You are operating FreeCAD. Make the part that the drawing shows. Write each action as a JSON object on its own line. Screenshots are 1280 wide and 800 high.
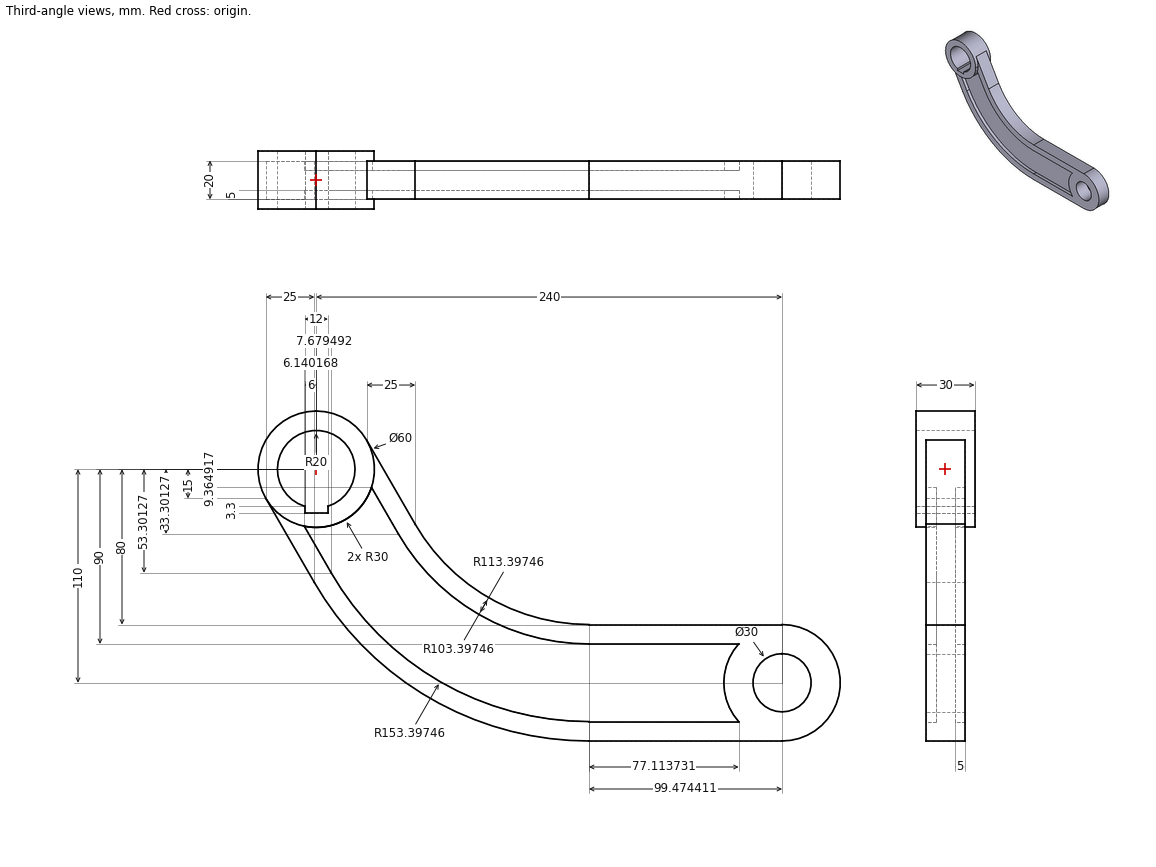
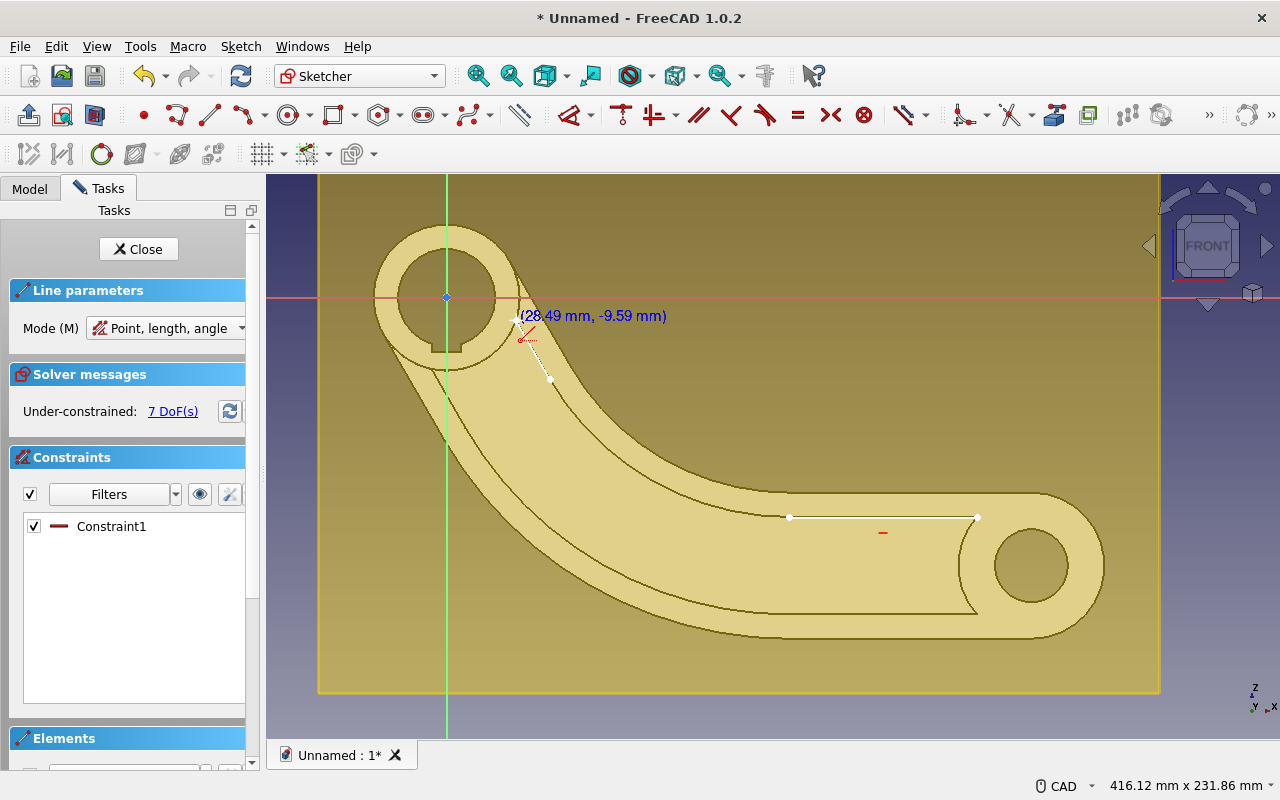
{"action": "left_click", "coordinate": [432, 369]}
{"action": "left_click", "coordinate": [465, 428]}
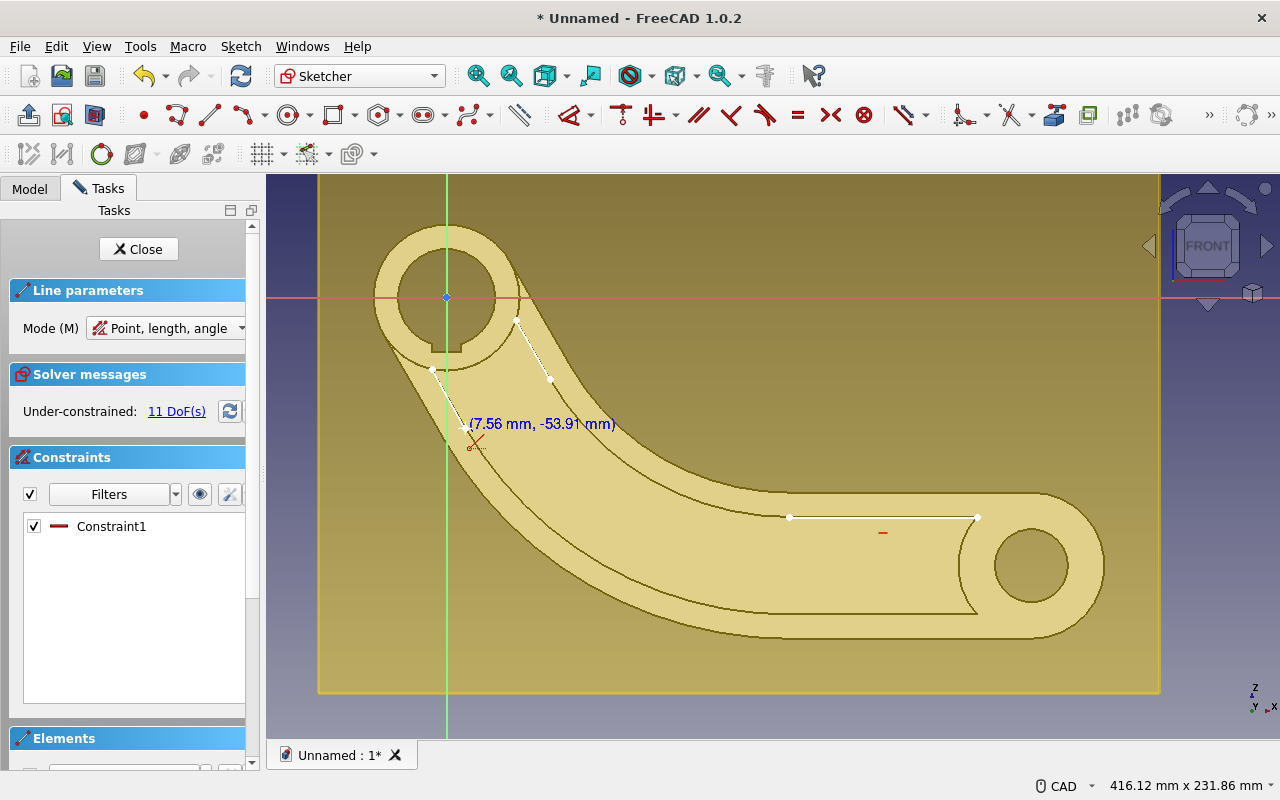
{"action": "left_click", "coordinate": [789, 614]}
{"action": "left_click", "coordinate": [977, 614]}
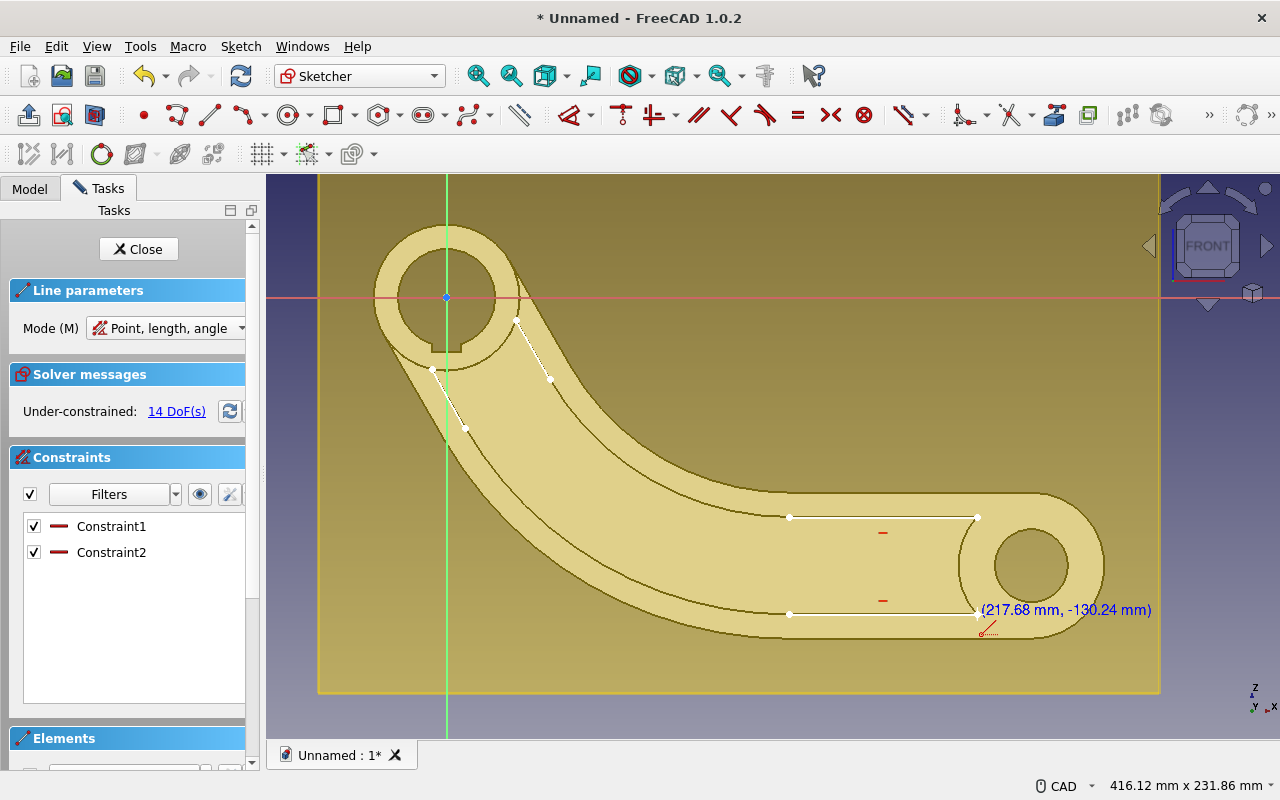
{"action": "left_click", "coordinate": [242, 116]}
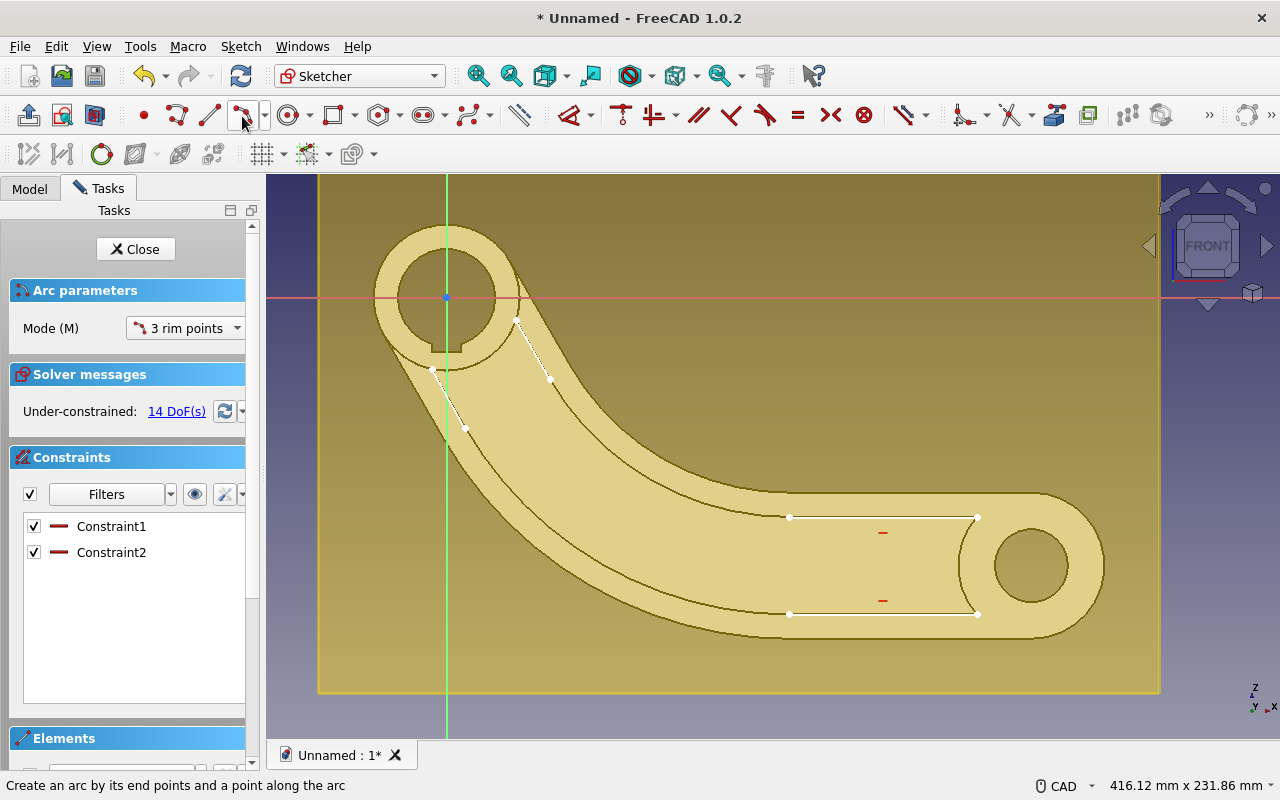
{"action": "left_click", "coordinate": [789, 518]}
{"action": "left_click", "coordinate": [550, 380]}
{"action": "left_click", "coordinate": [651, 480]}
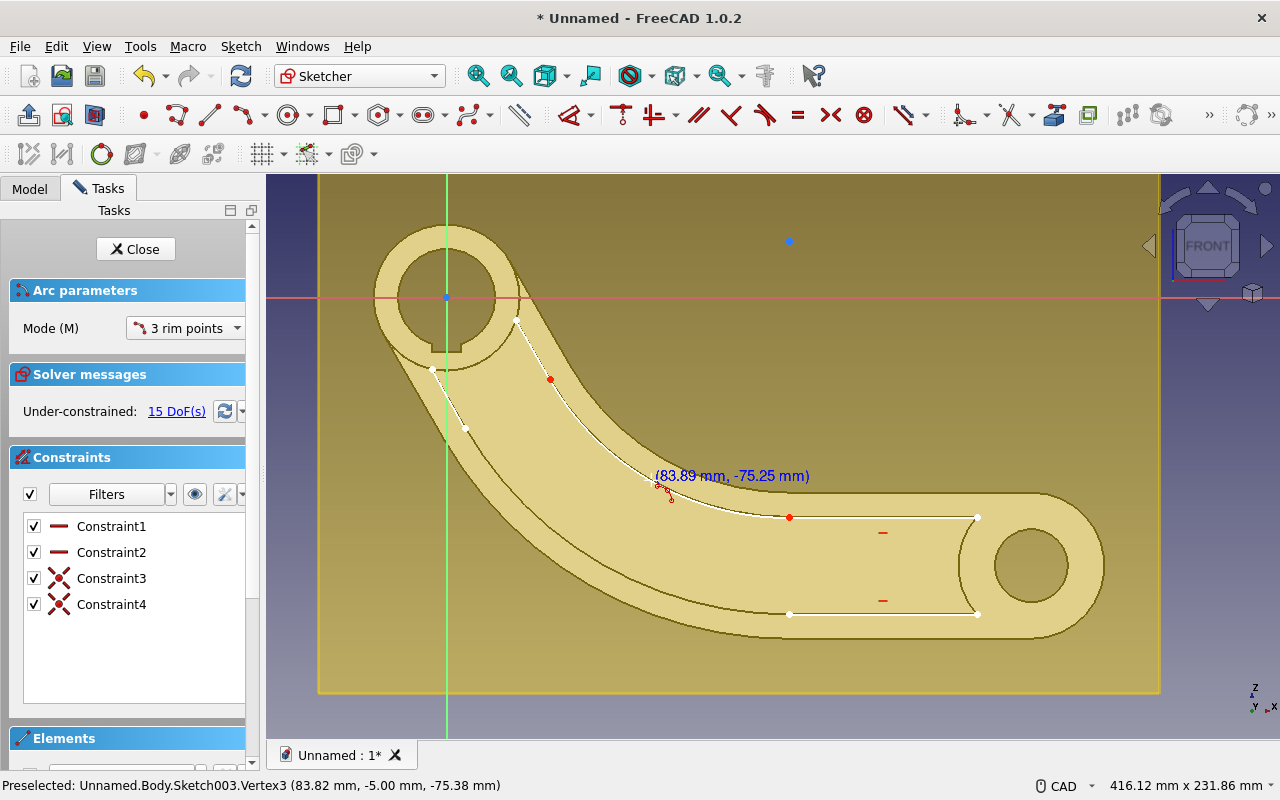
{"action": "left_click", "coordinate": [516, 321]}
{"action": "left_click", "coordinate": [432, 370]}
{"action": "left_click", "coordinate": [483, 361]}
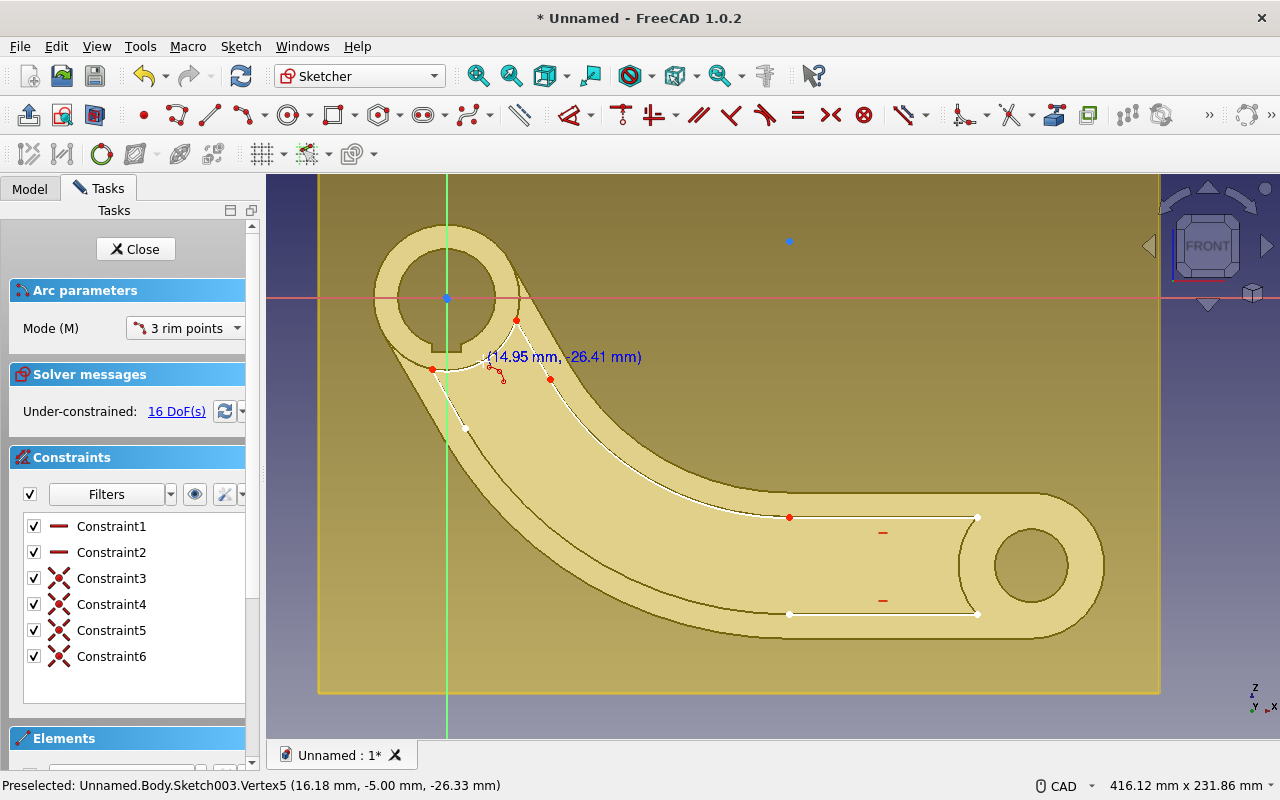
{"action": "left_click", "coordinate": [465, 429]}
{"action": "left_click", "coordinate": [789, 615]}
{"action": "left_click", "coordinate": [602, 564]}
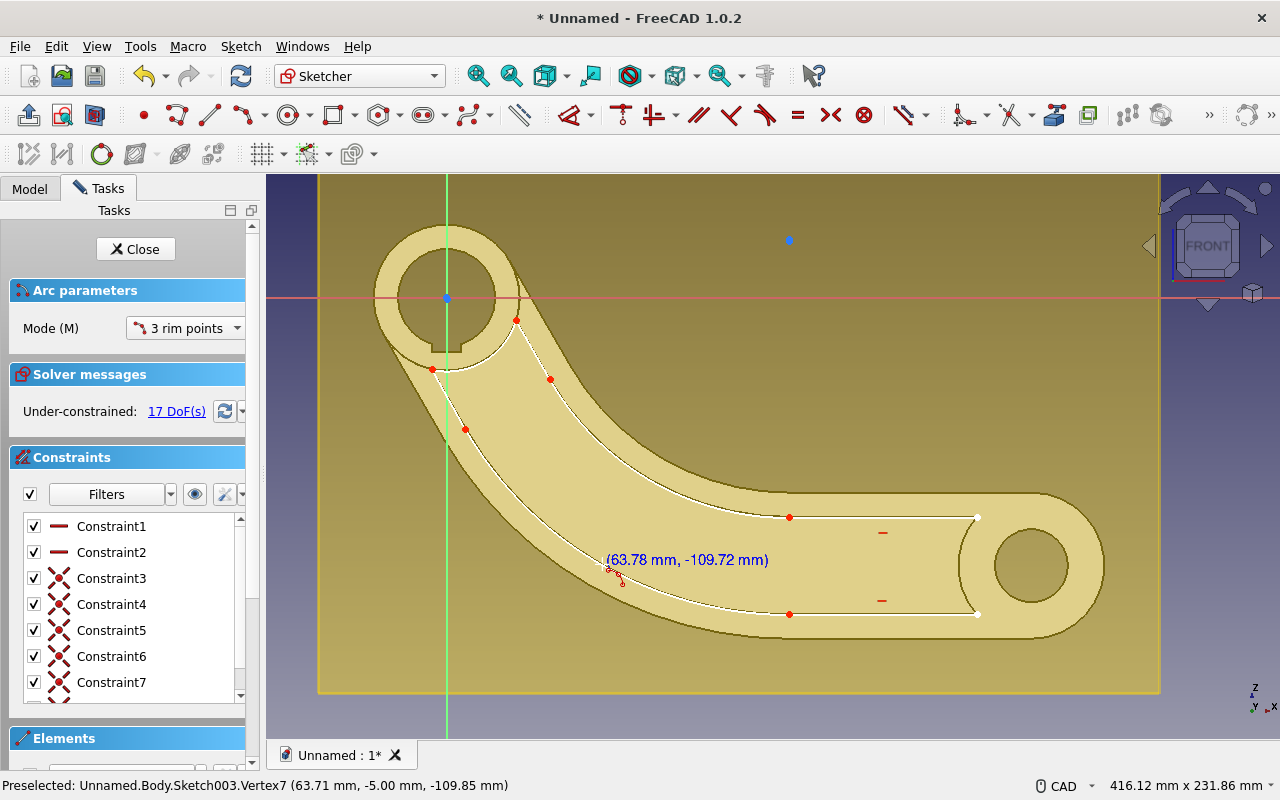
{"action": "left_click", "coordinate": [977, 615]}
{"action": "left_click", "coordinate": [977, 518]}
{"action": "left_click", "coordinate": [958, 566]}
{"action": "key", "text": "Escape"}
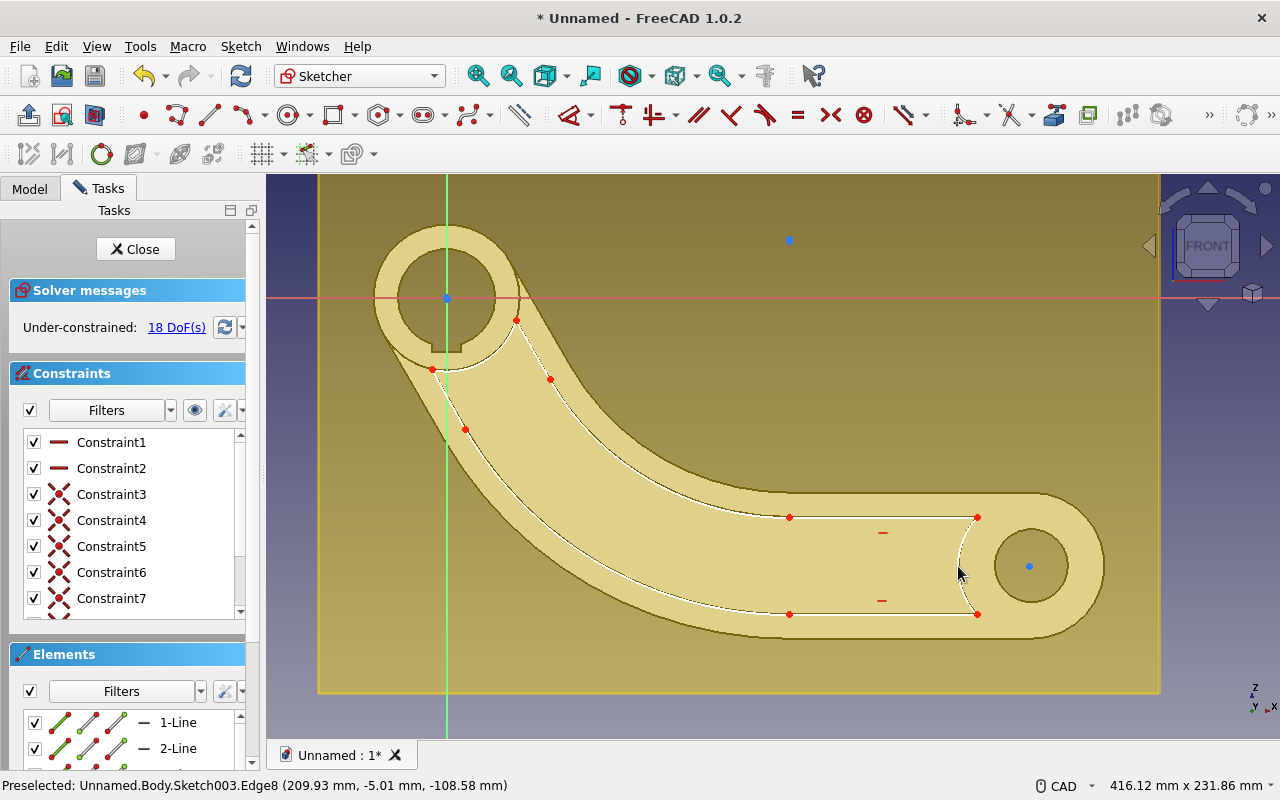
{"action": "left_click", "coordinate": [540, 362]}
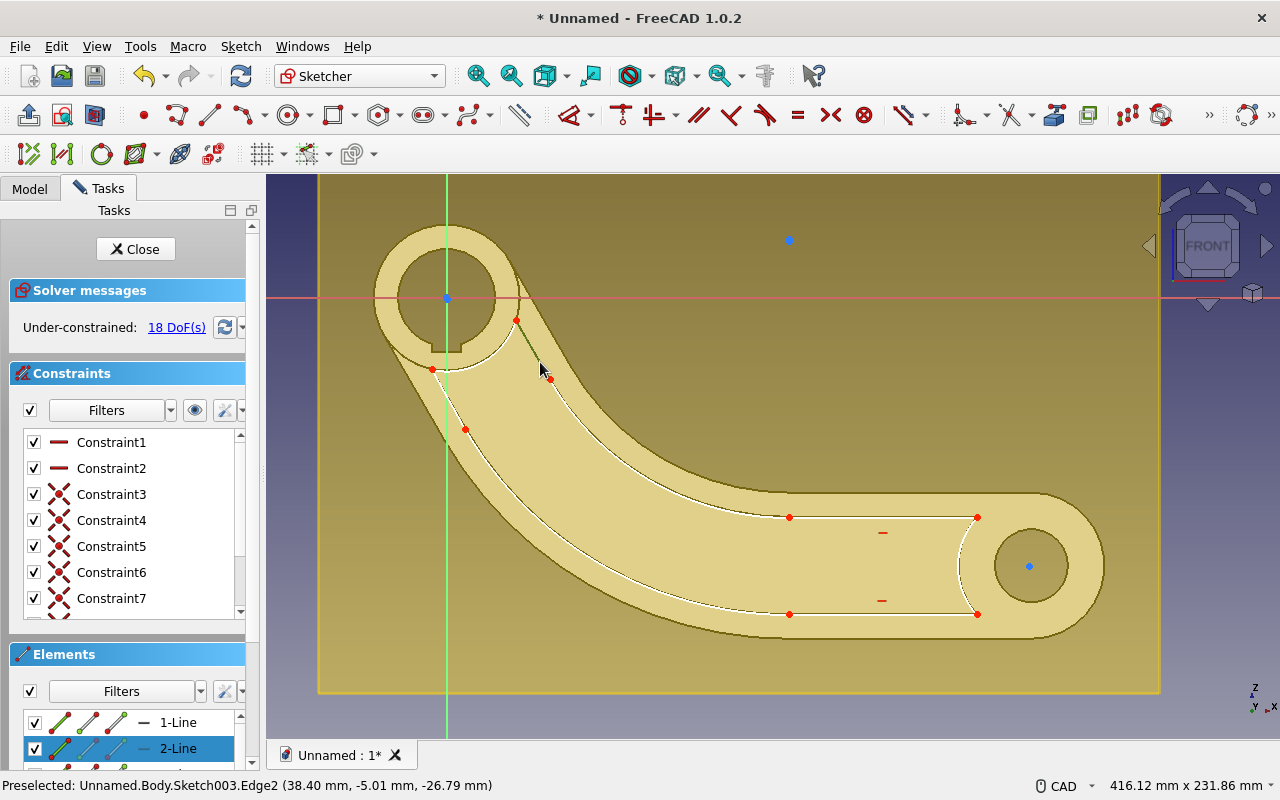
{"action": "left_click", "coordinate": [604, 447]}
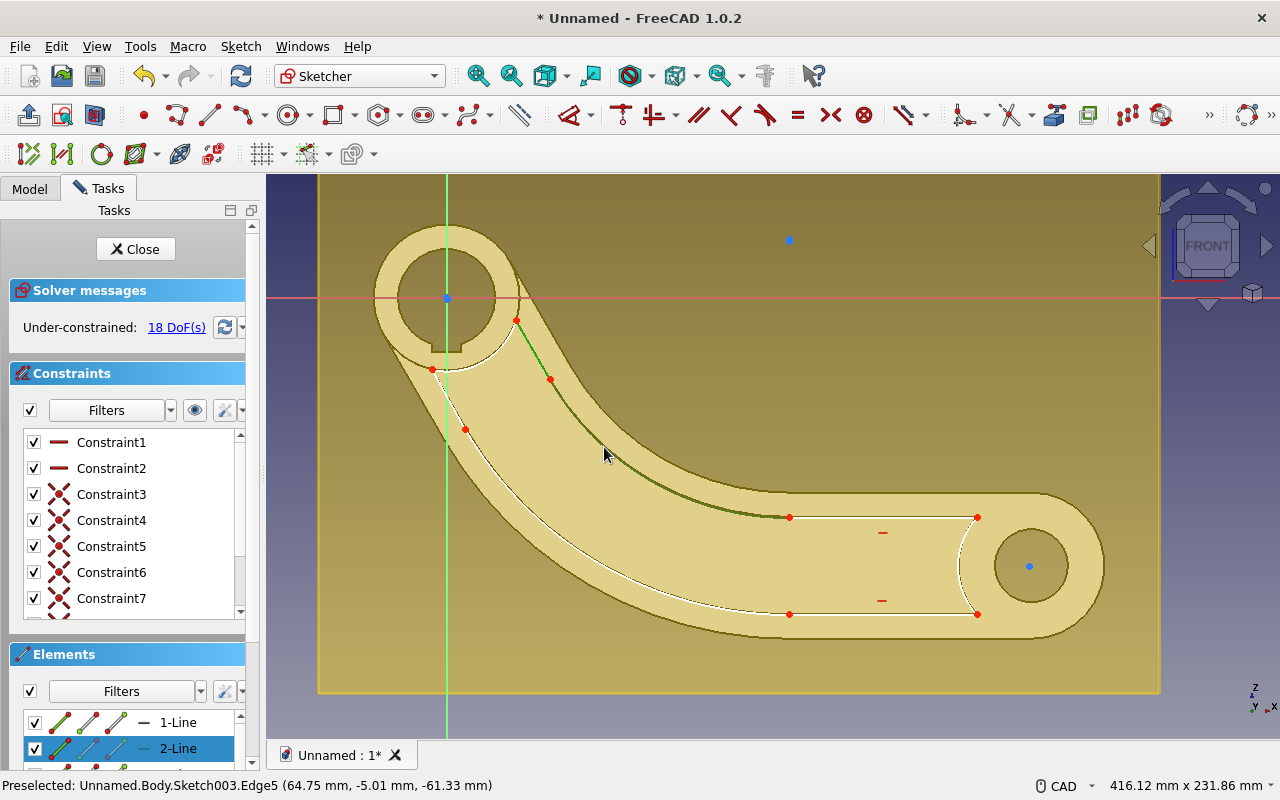
{"action": "left_click", "coordinate": [765, 116]}